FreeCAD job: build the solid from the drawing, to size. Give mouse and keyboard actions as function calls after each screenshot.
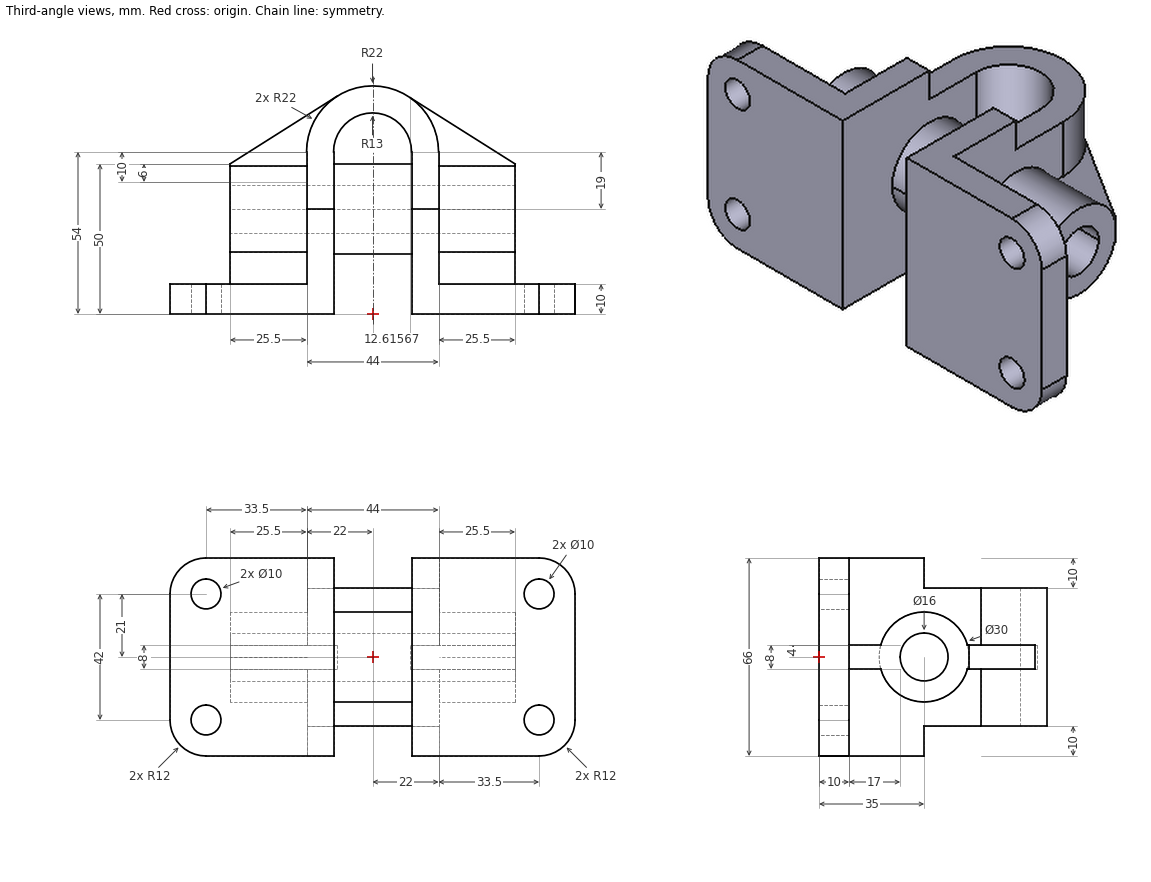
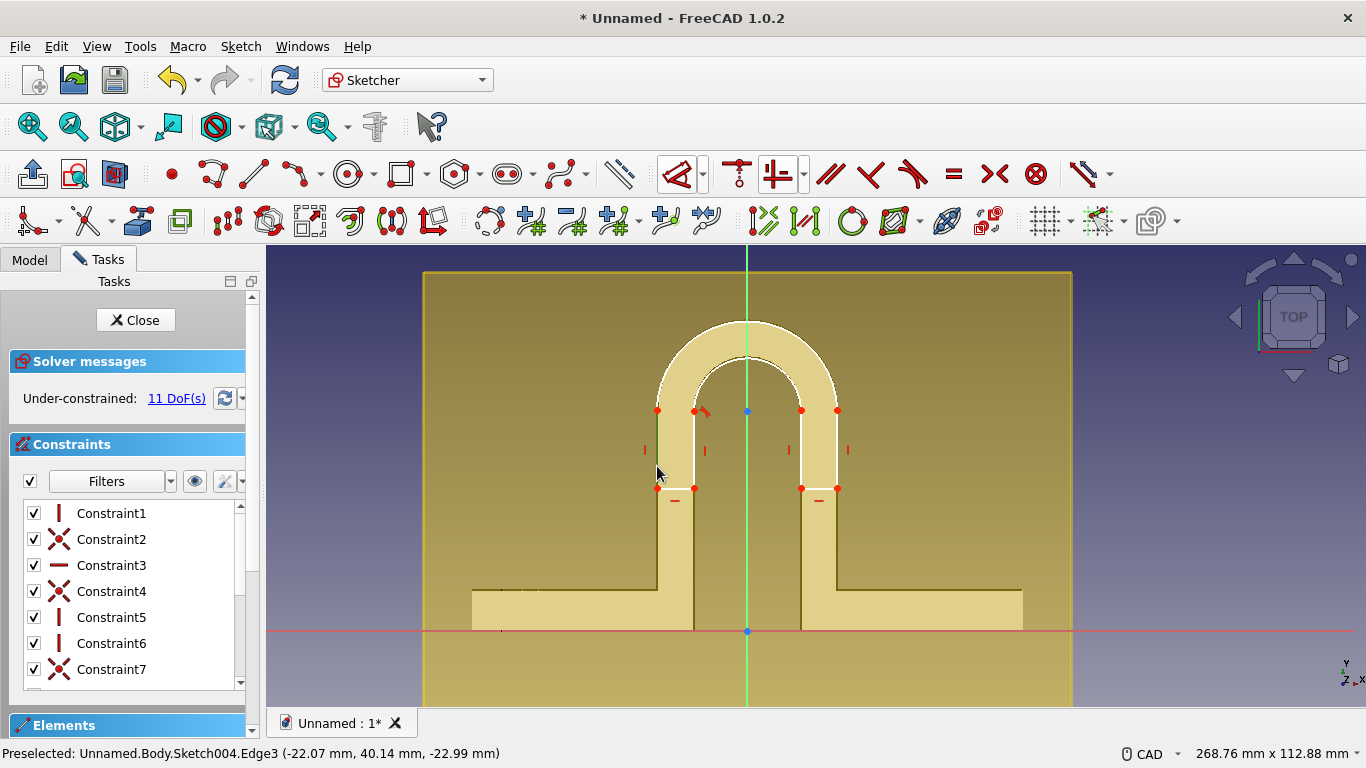
click(800, 339)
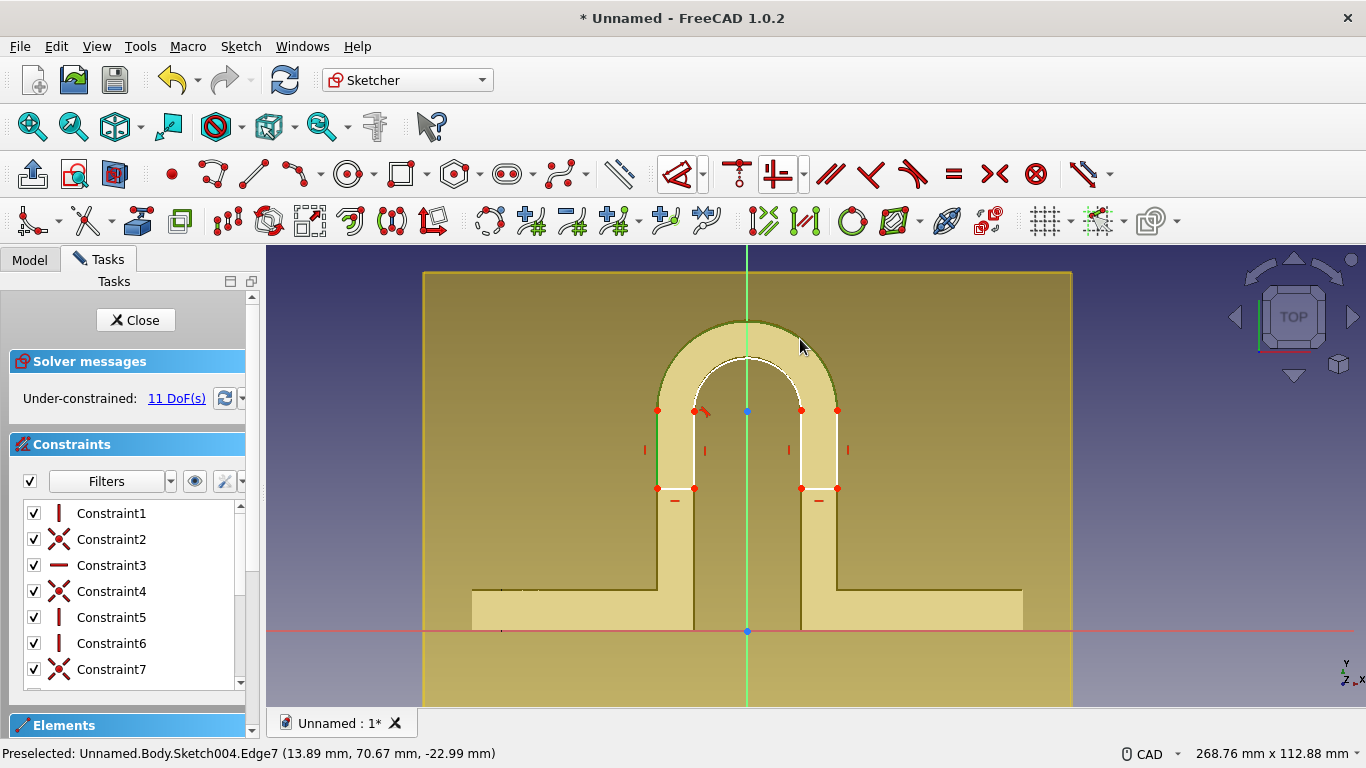
click(913, 174)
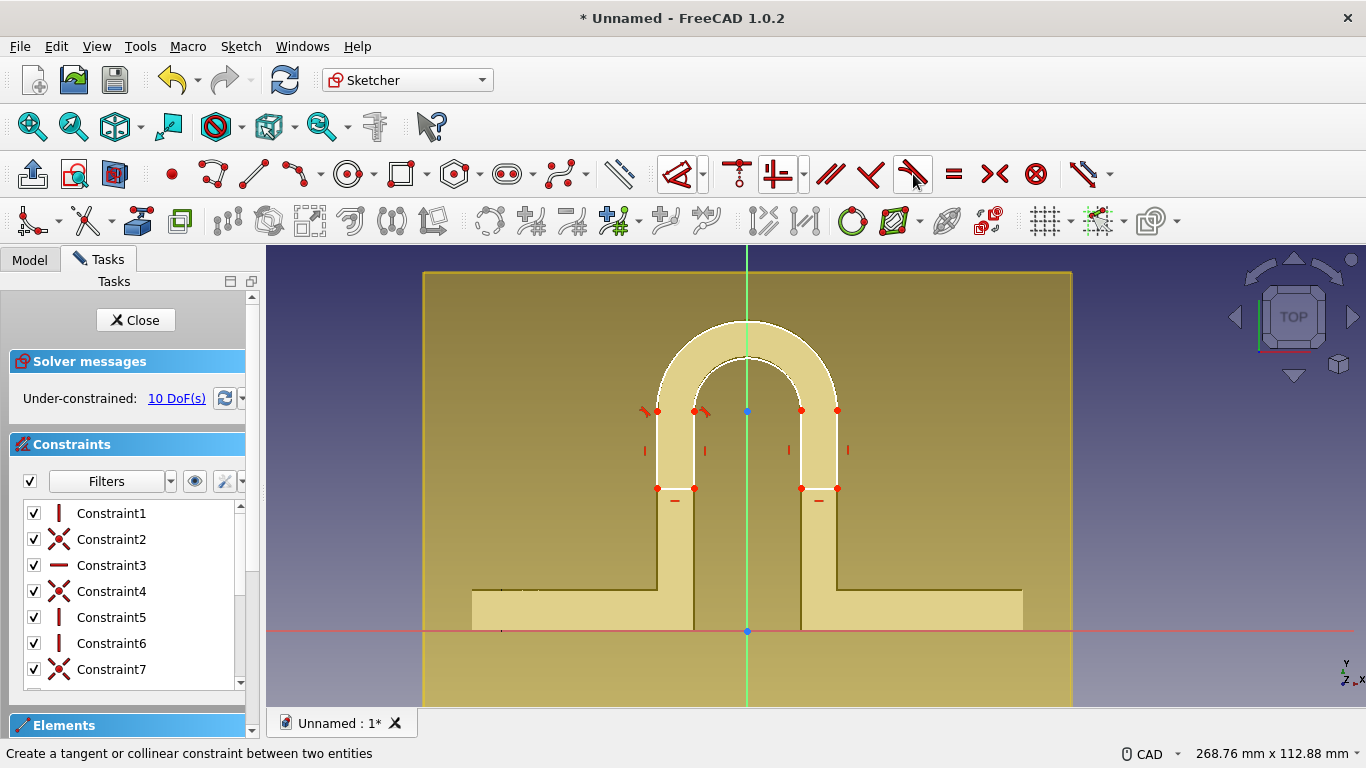
click(837, 434)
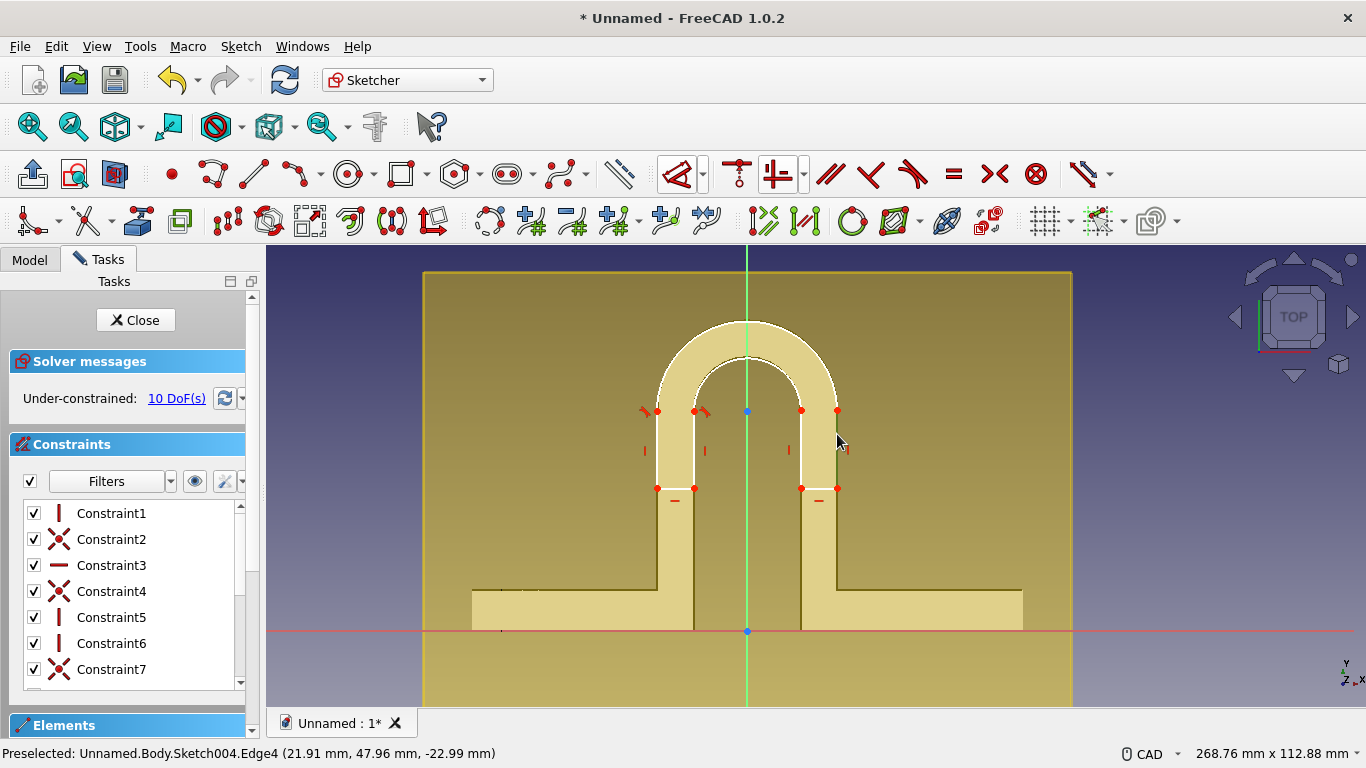
click(800, 339)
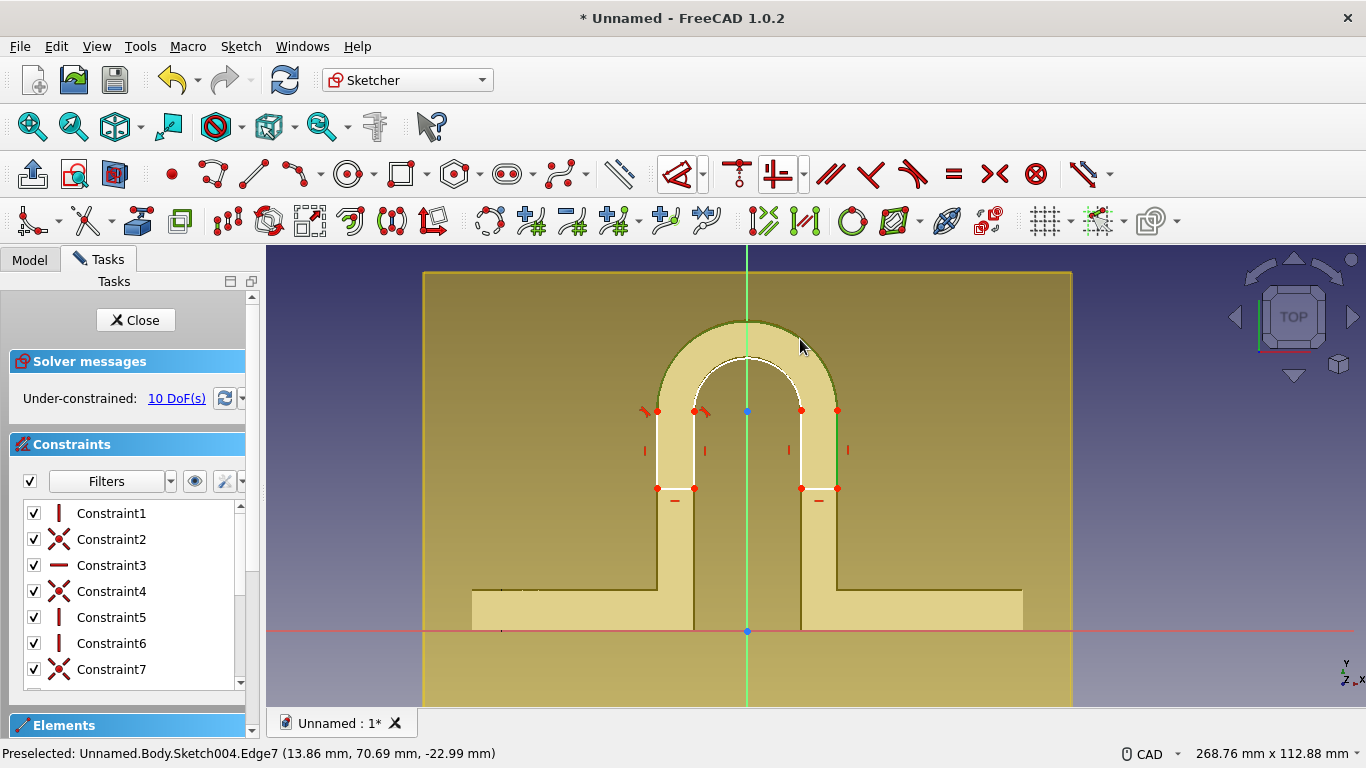
click(913, 174)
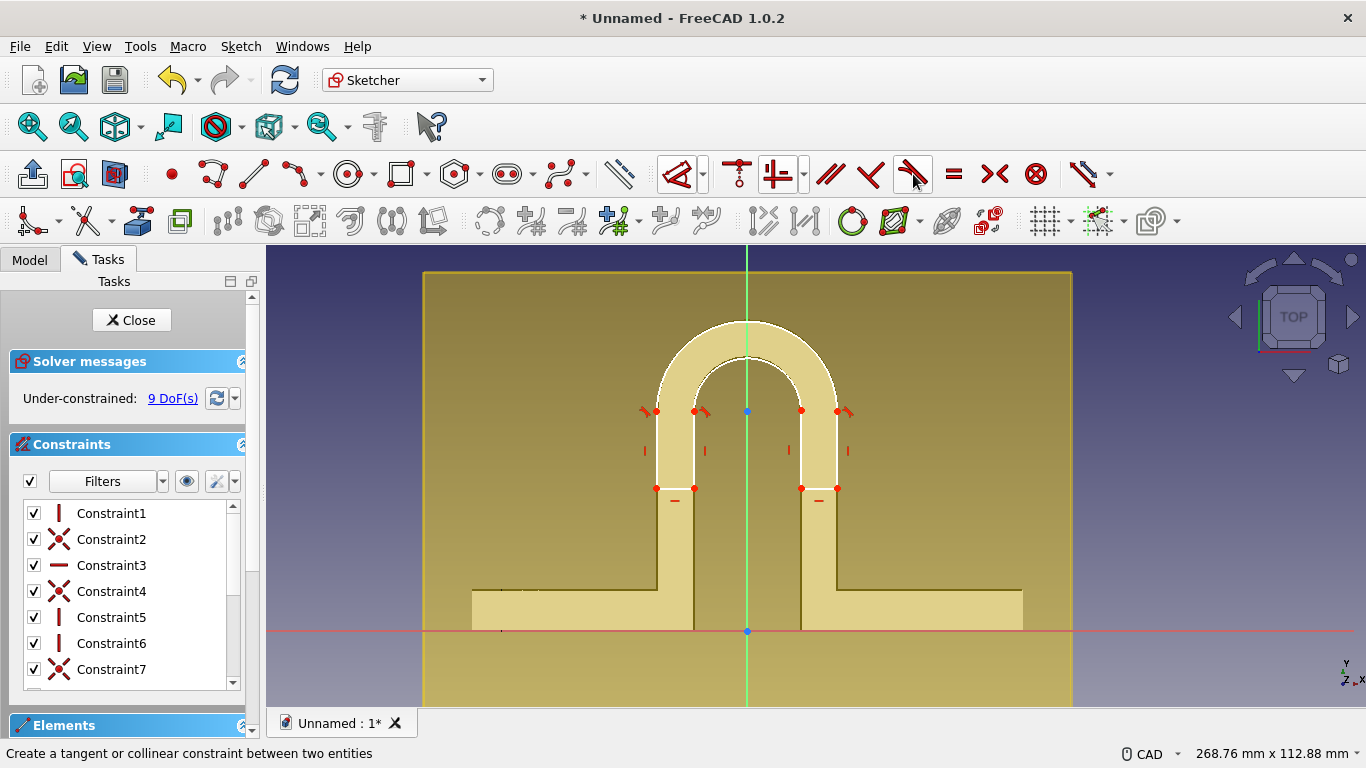
click(801, 466)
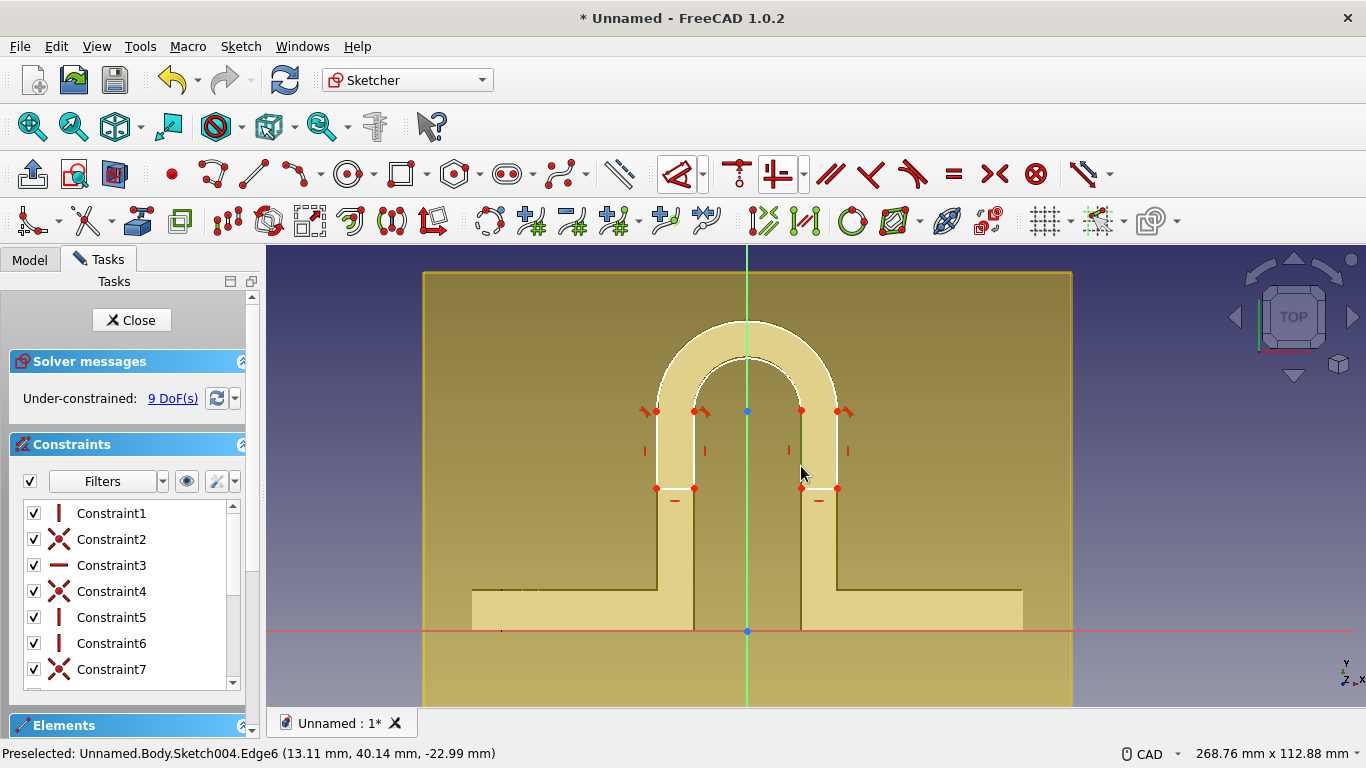
click(778, 368)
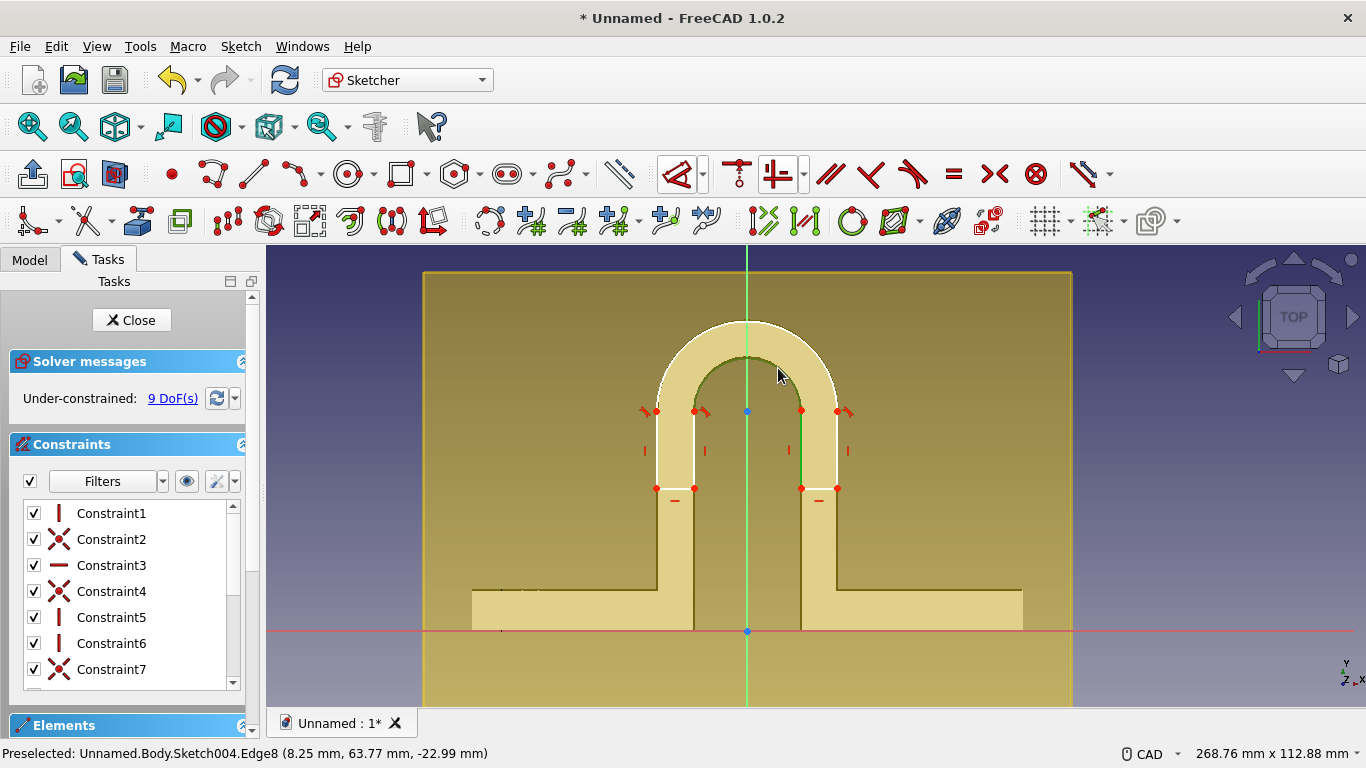
click(913, 174)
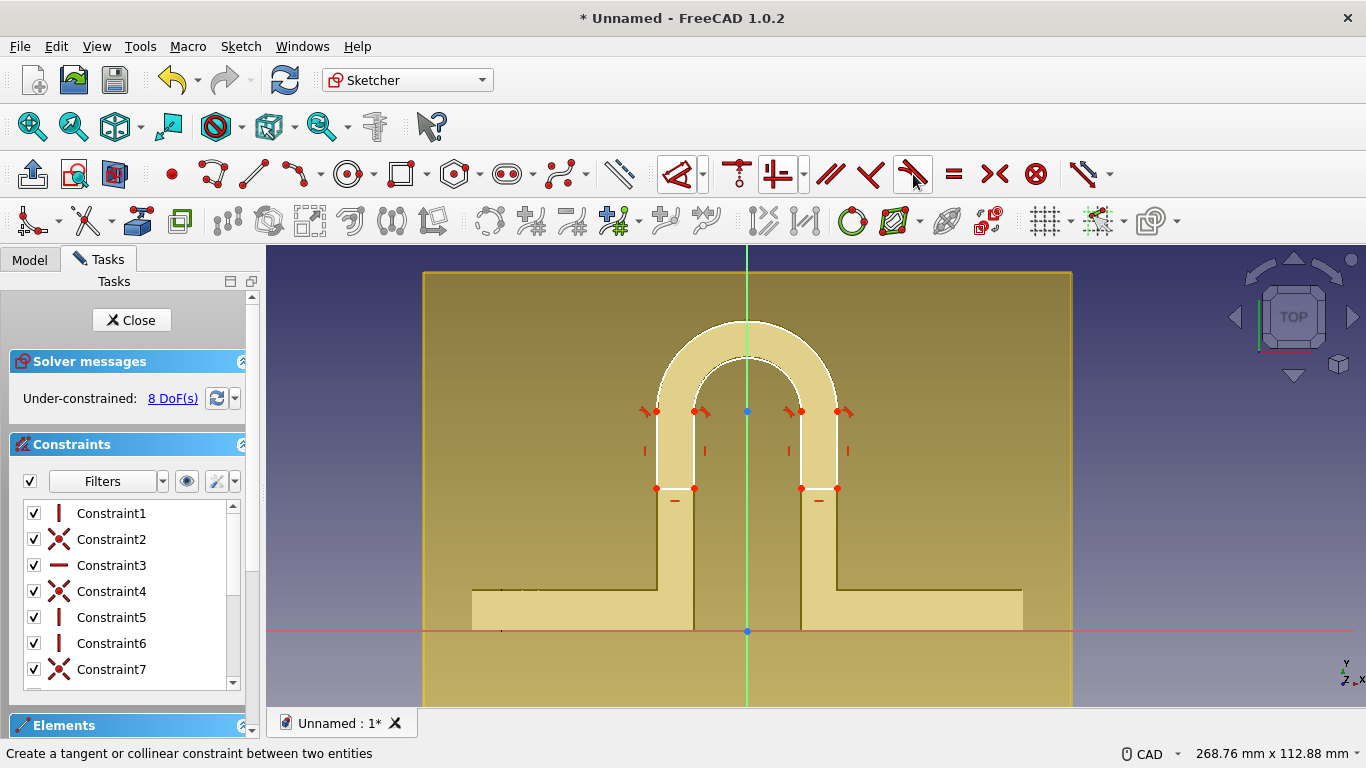
click(800, 339)